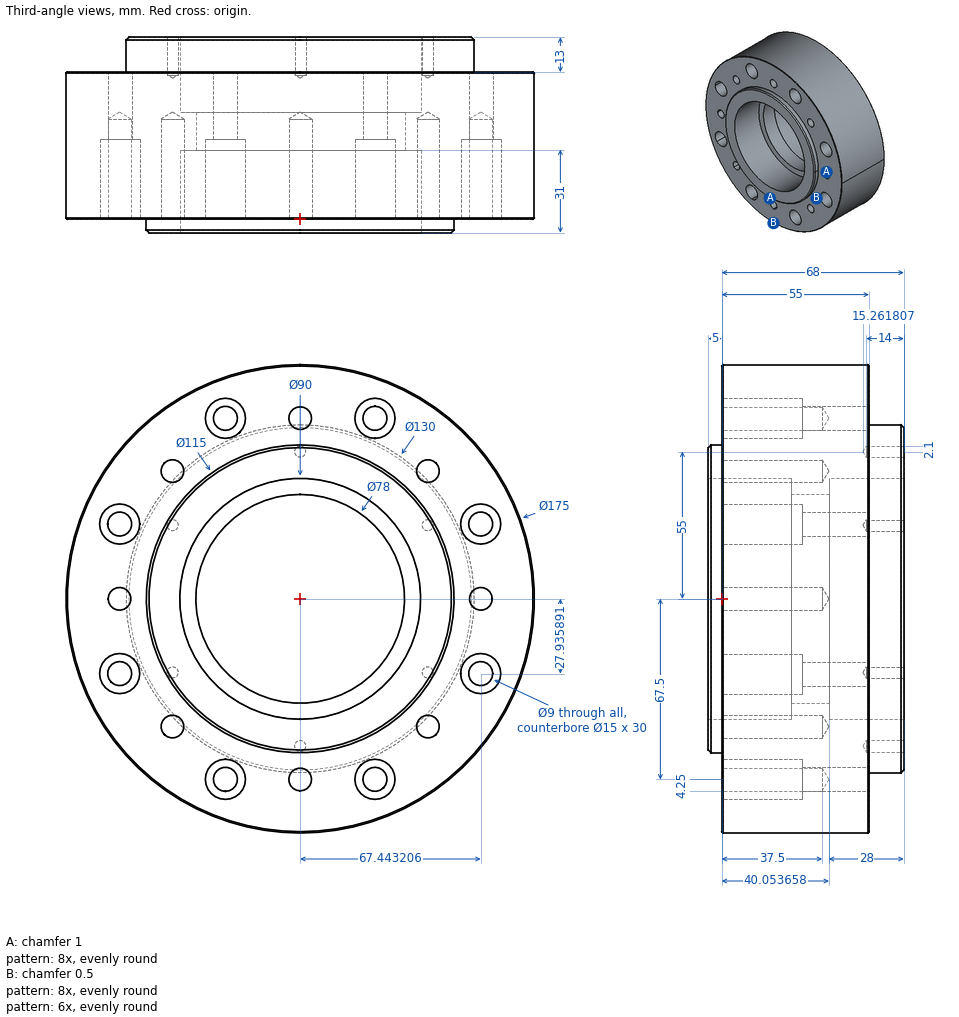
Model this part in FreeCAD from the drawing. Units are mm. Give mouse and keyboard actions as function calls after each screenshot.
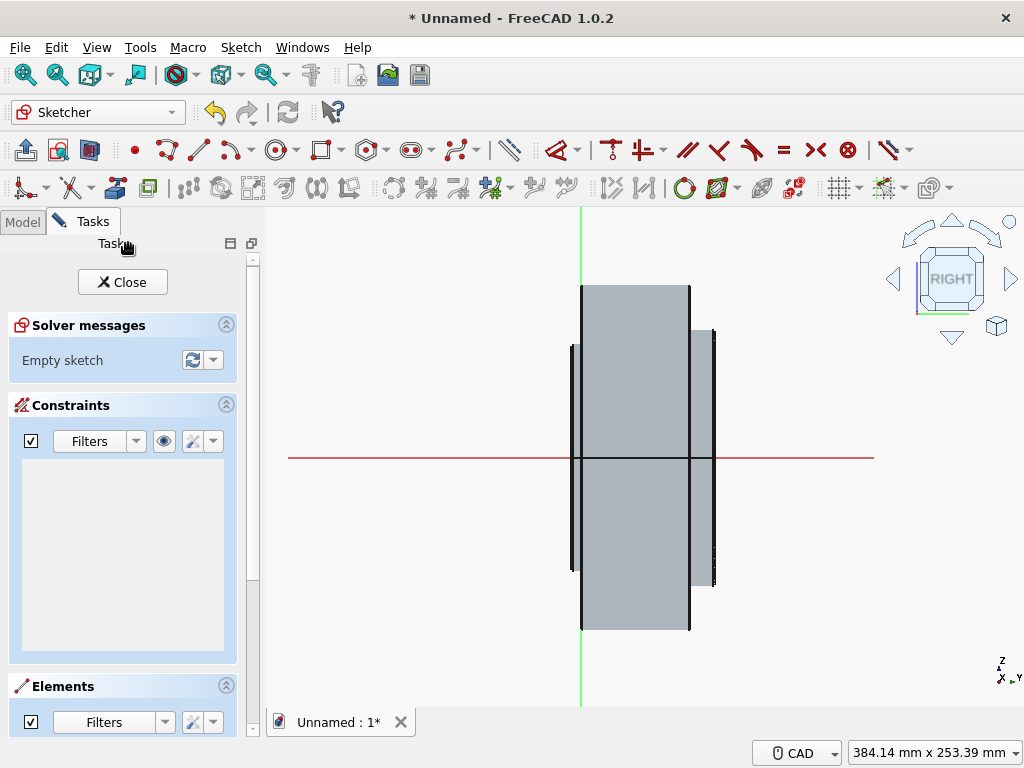
key(q)
key(s)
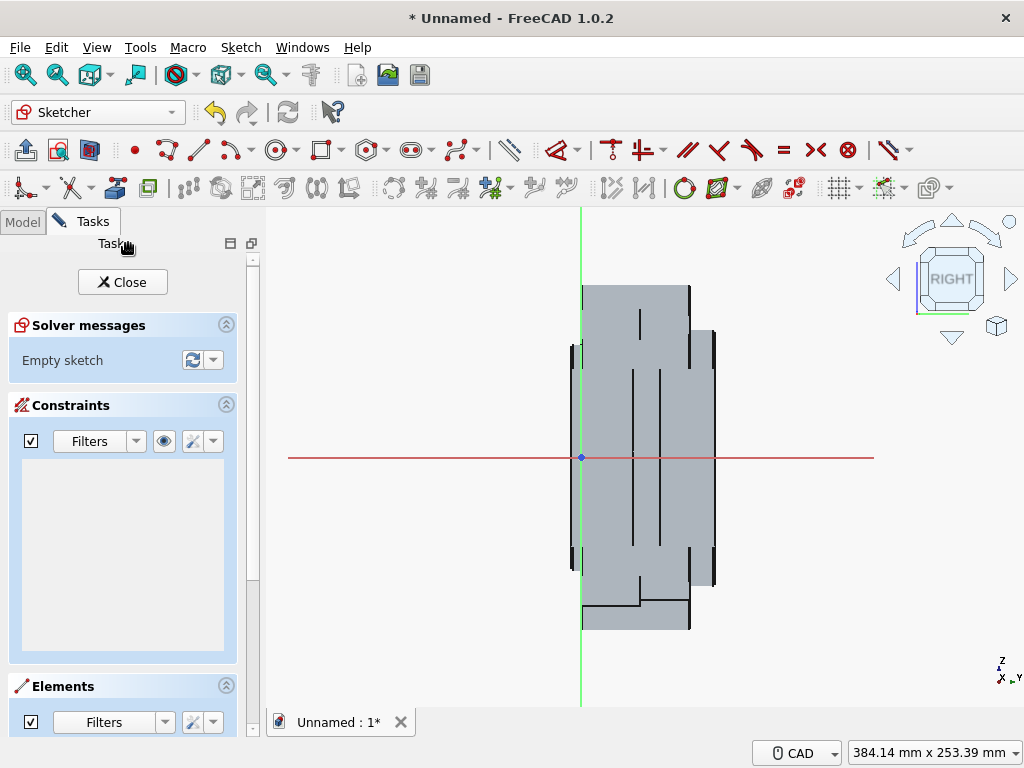
scroll(686, 587, up, 4)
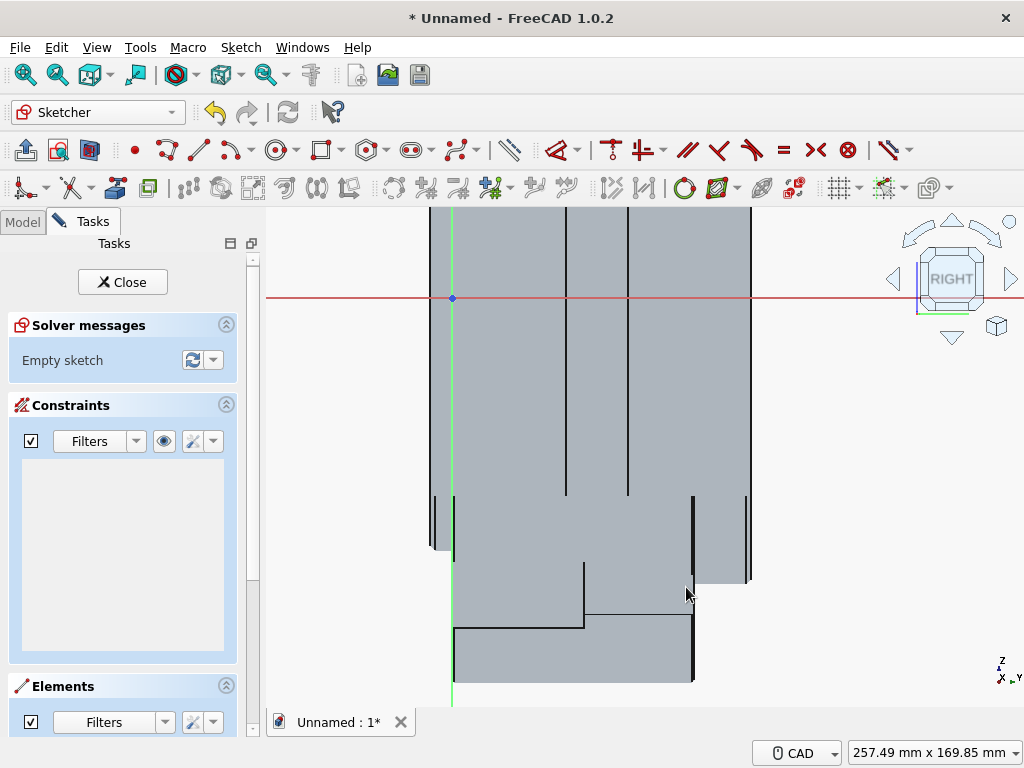
click(168, 150)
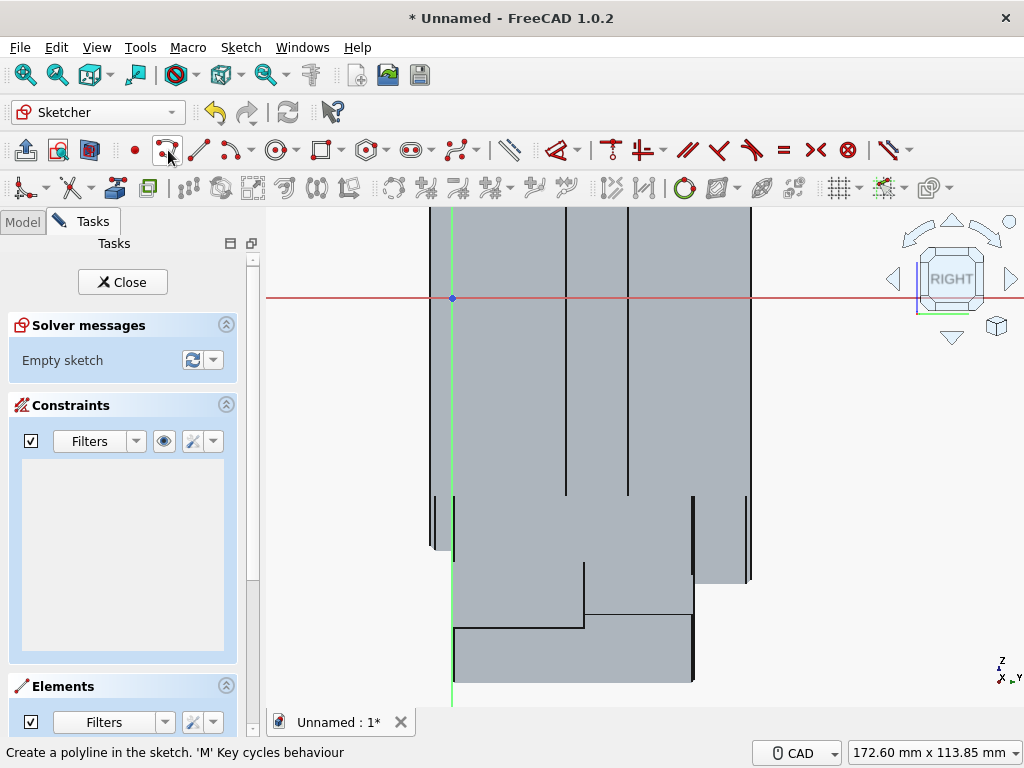
click(452, 595)
click(461, 614)
click(617, 614)
click(628, 595)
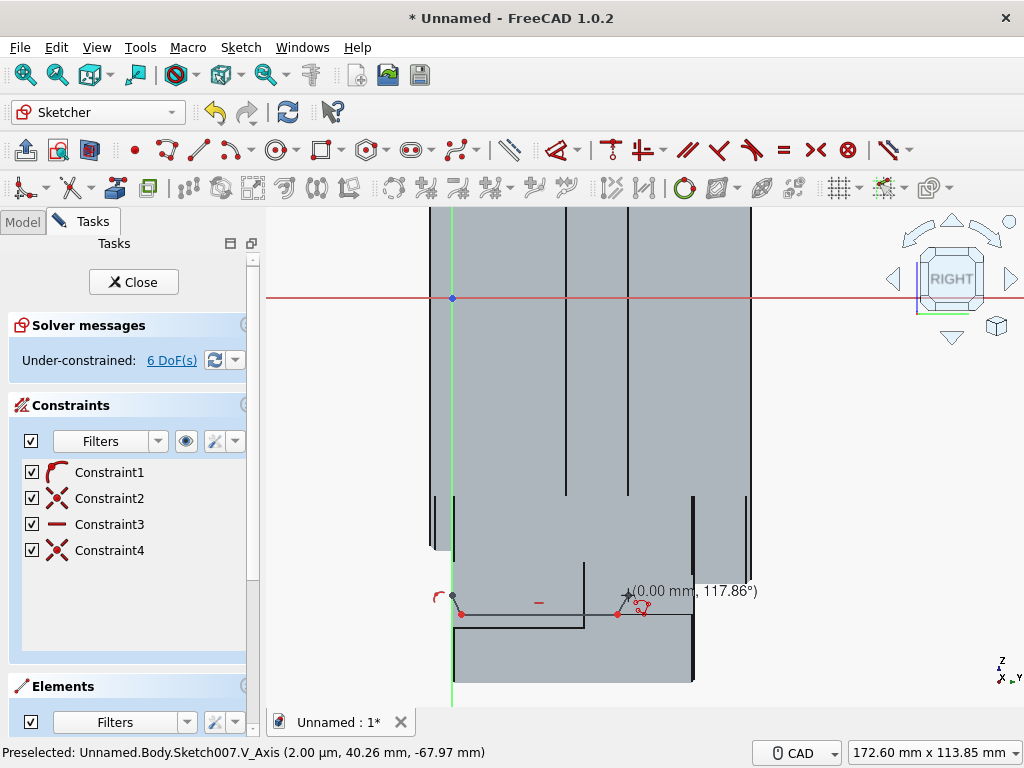
scroll(452, 595, up, 3)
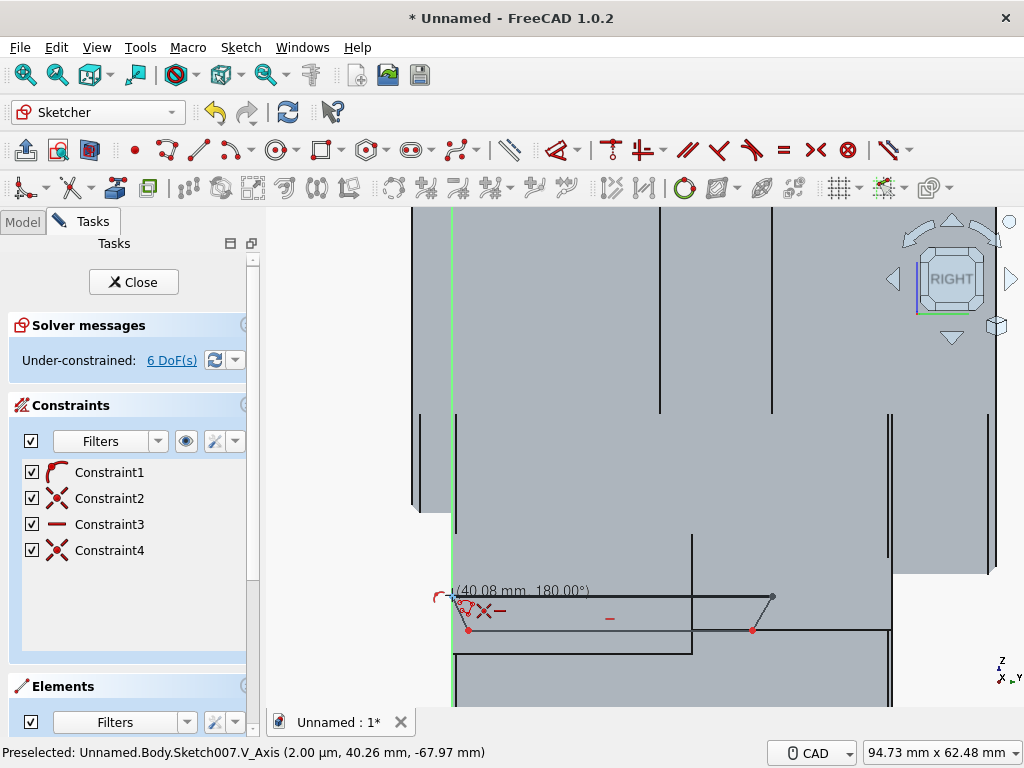
click(452, 596)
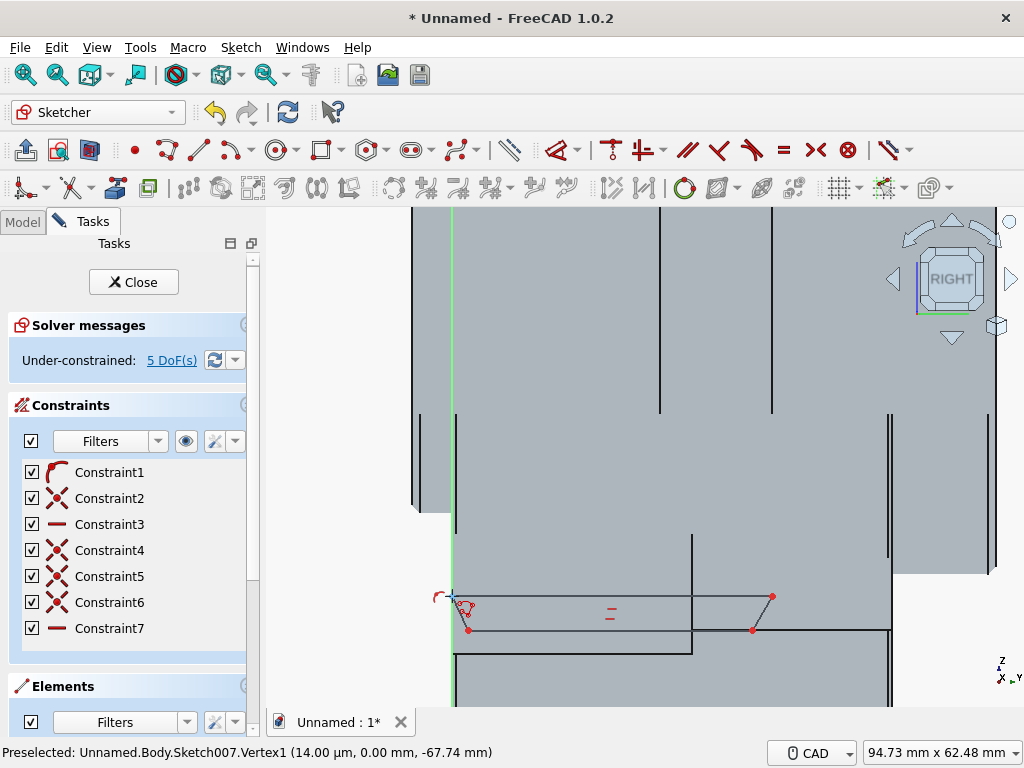
click(200, 150)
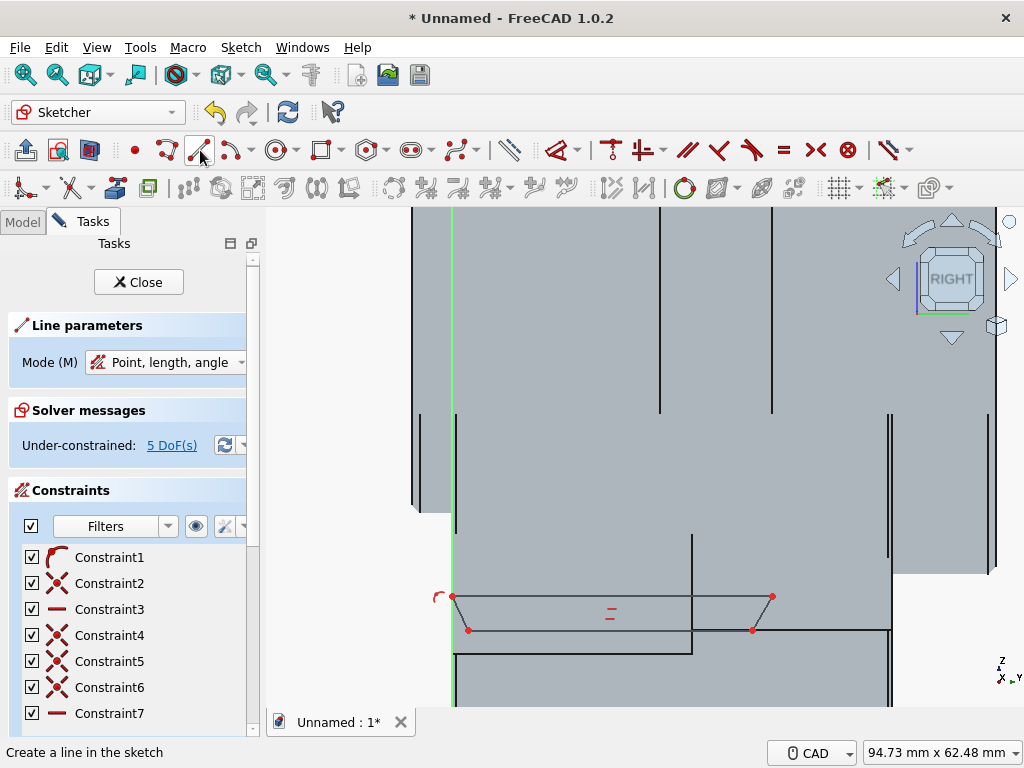
click(805, 594)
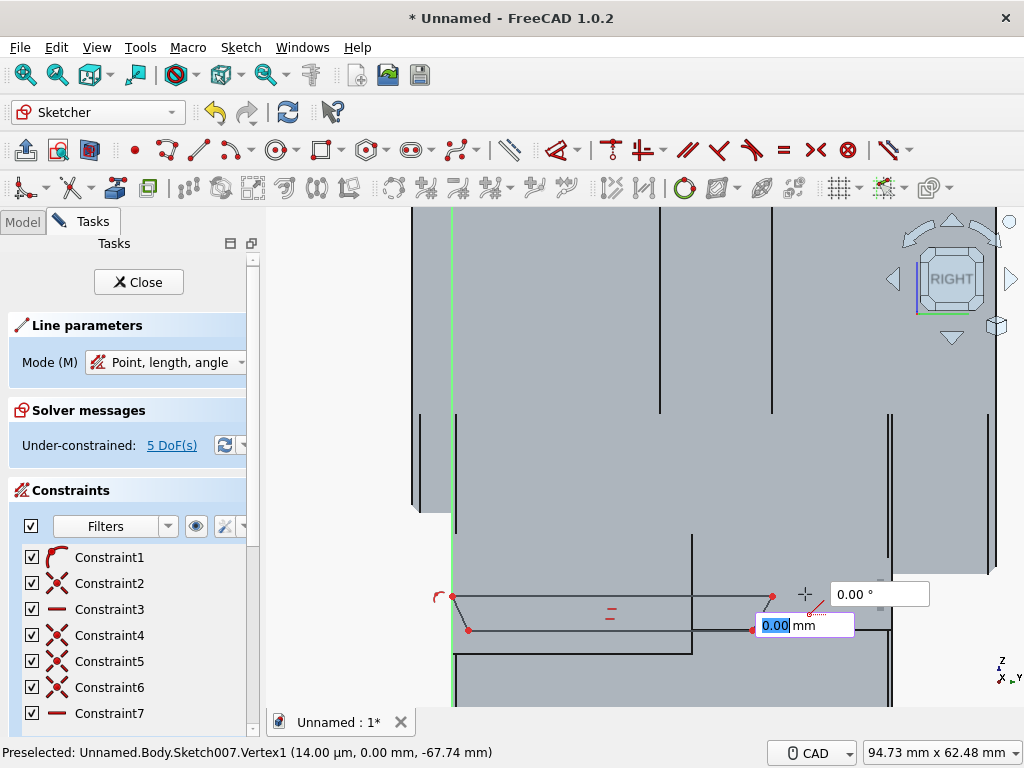
scroll(455, 598, down, 3)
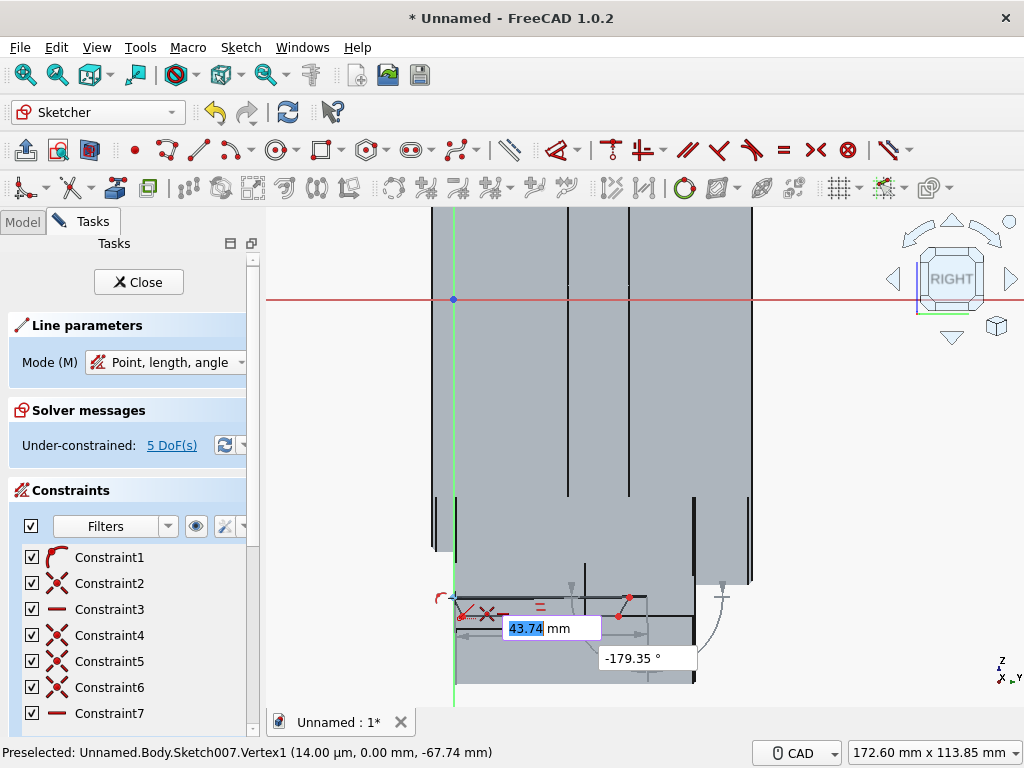
click(700, 596)
key(Escape)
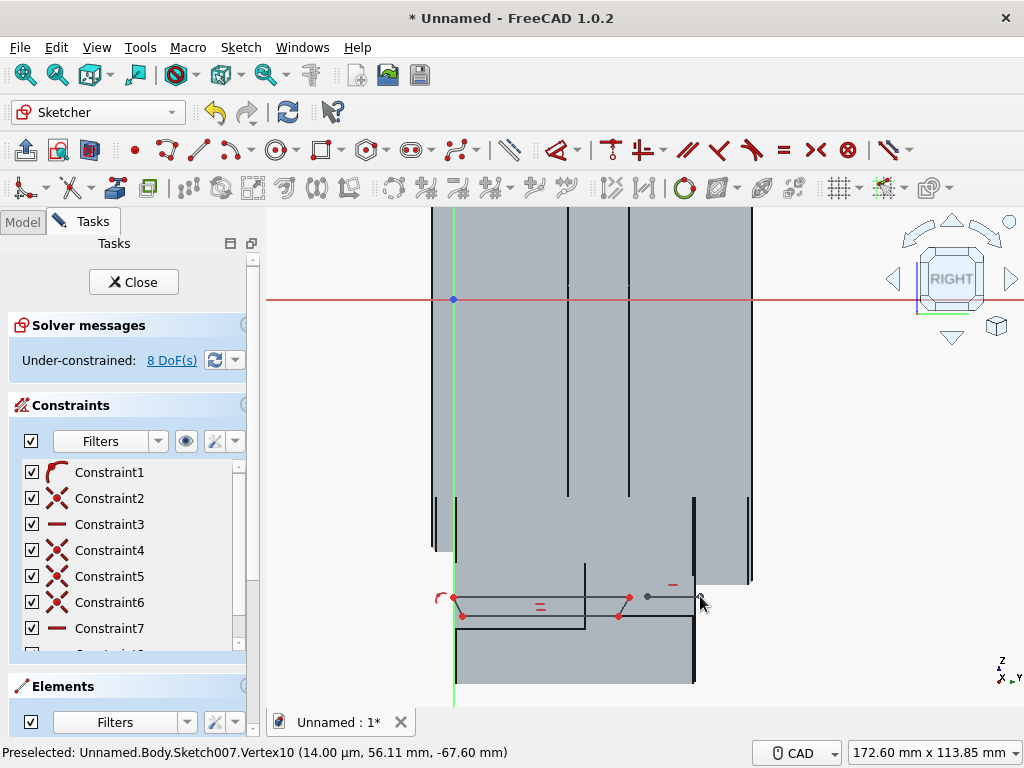
click(663, 597)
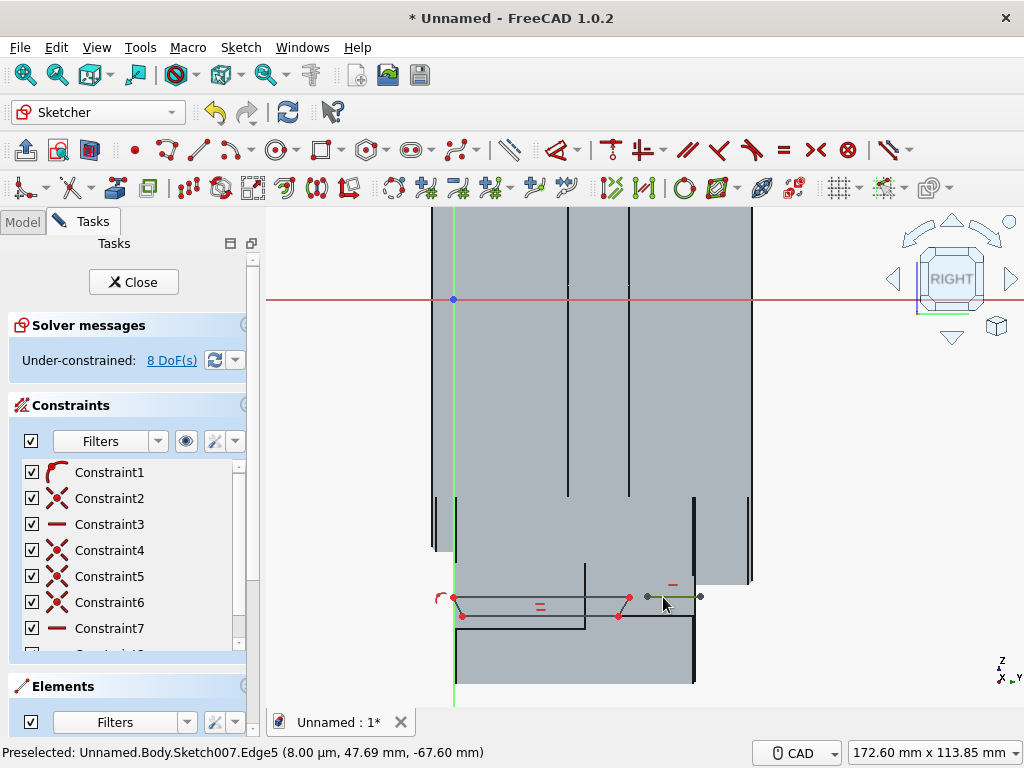
click(510, 150)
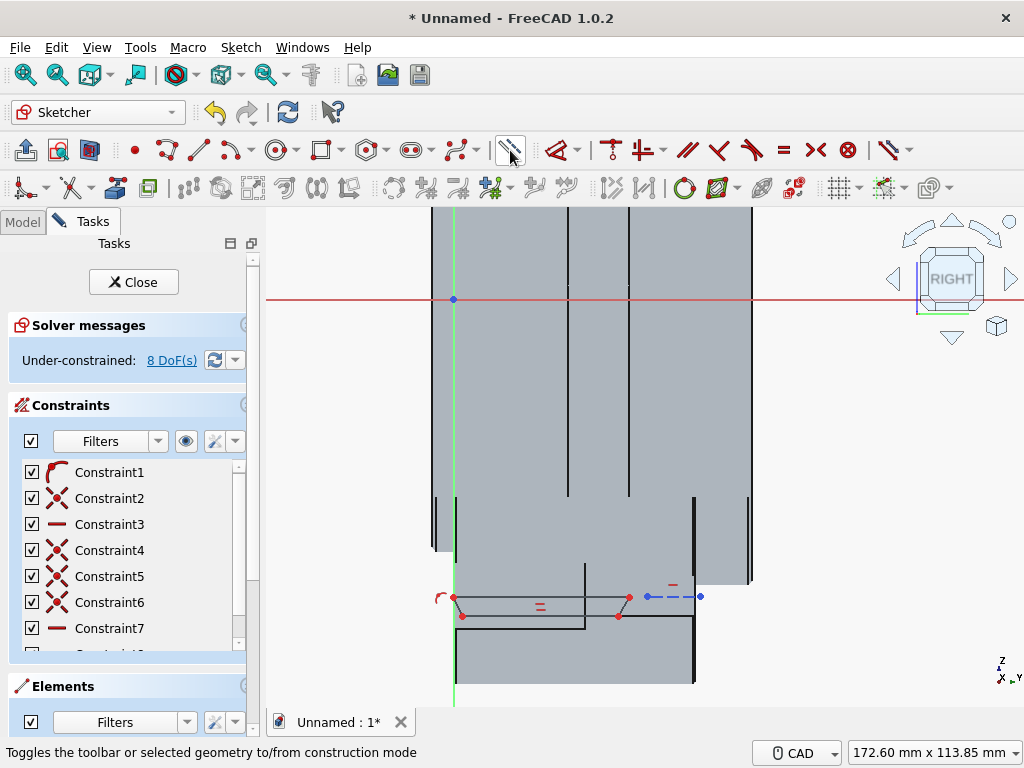
scroll(457, 605, up, 3)